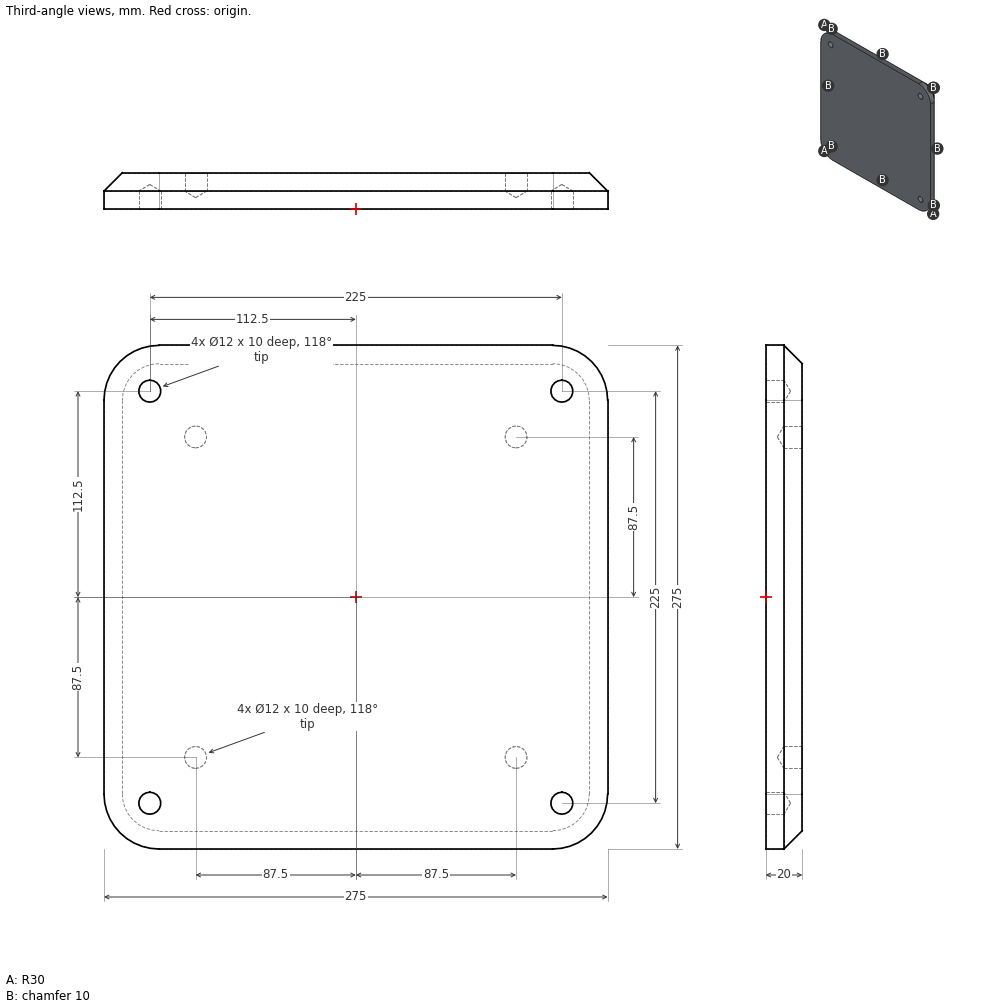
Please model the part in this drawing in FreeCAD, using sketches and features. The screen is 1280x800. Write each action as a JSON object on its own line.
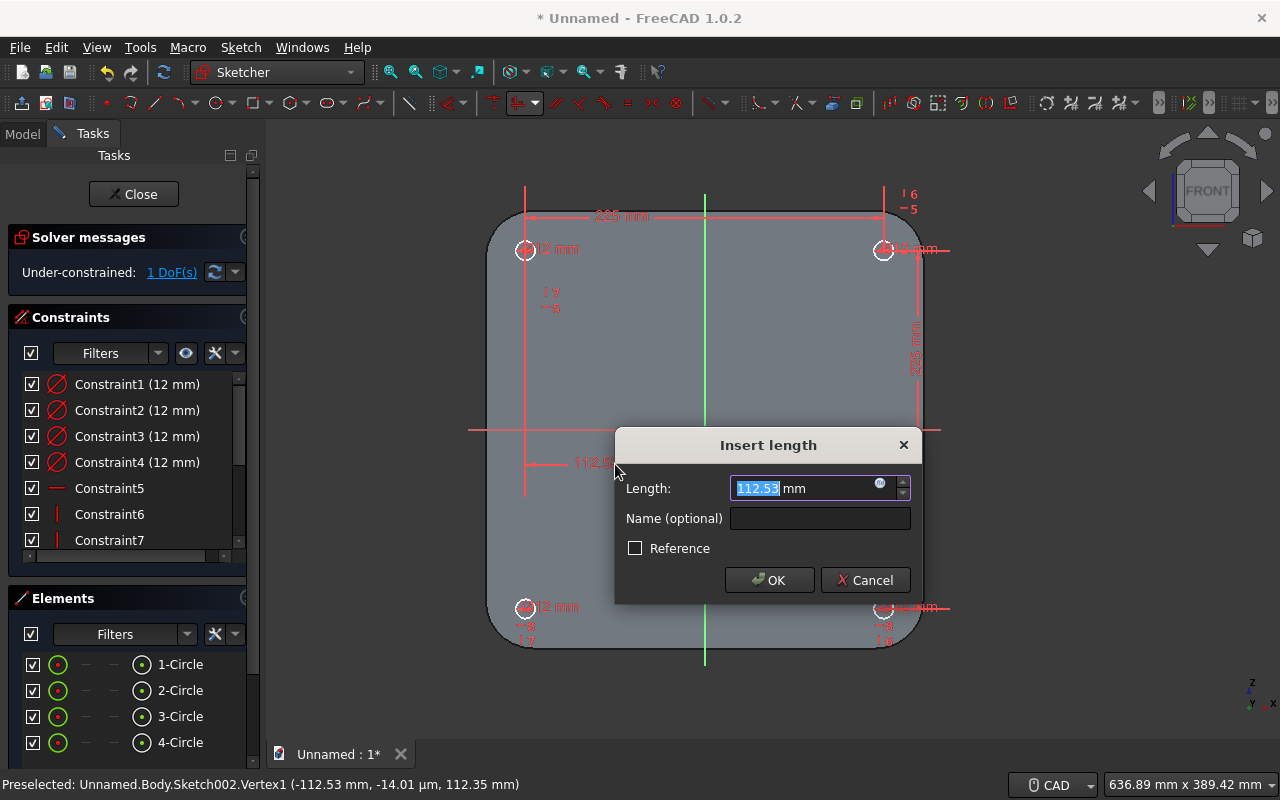
{"action": "type", "text": "112.5"}
{"action": "key", "text": "Return"}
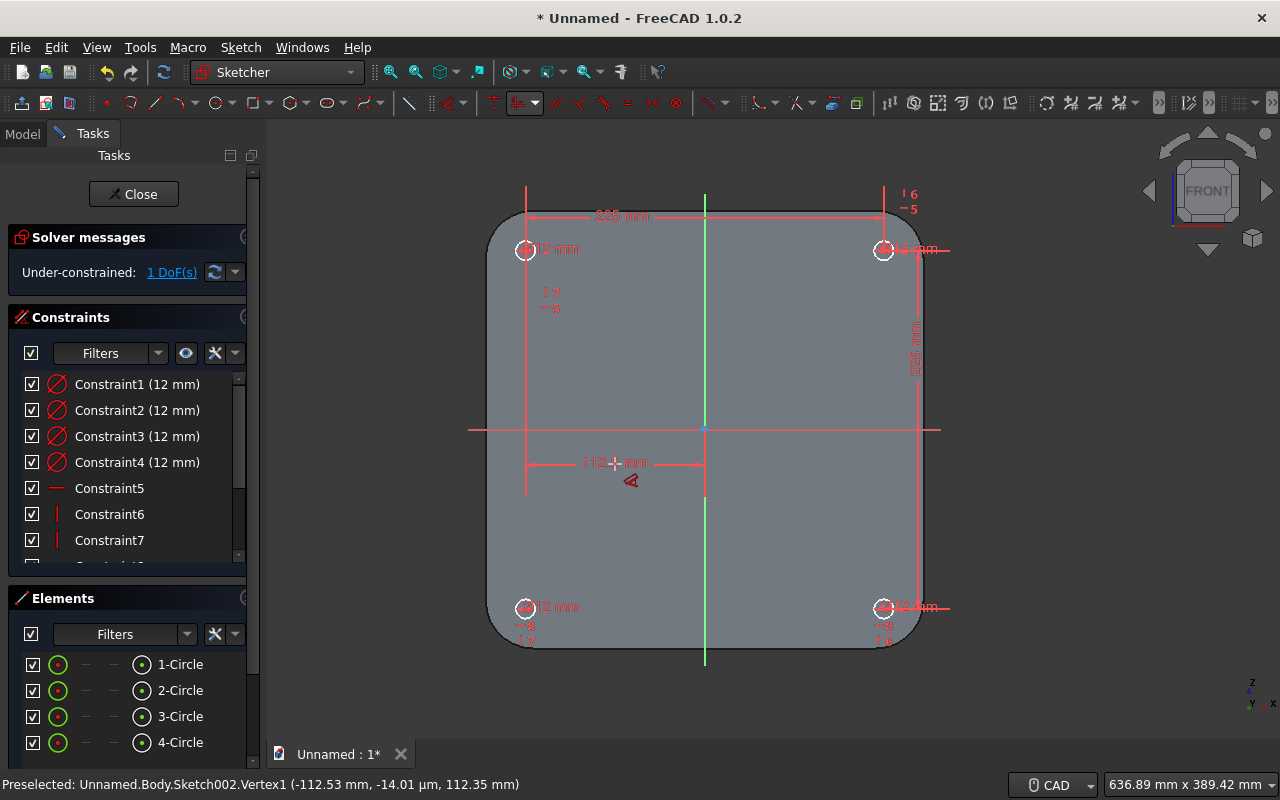
{"action": "left_click", "coordinate": [526, 251]}
{"action": "left_click", "coordinate": [492, 340]}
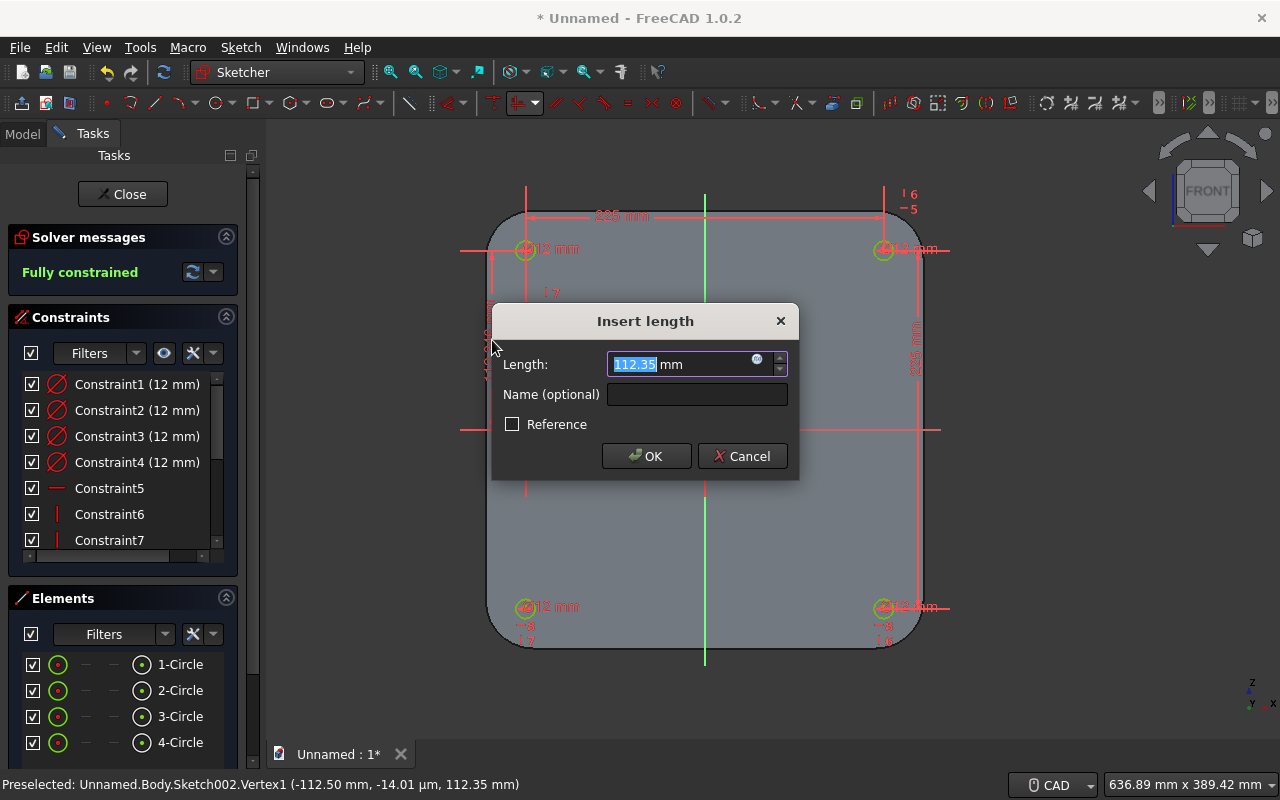
{"action": "type", "text": "112.5"}
{"action": "key", "text": "Return"}
{"action": "key", "text": "Escape"}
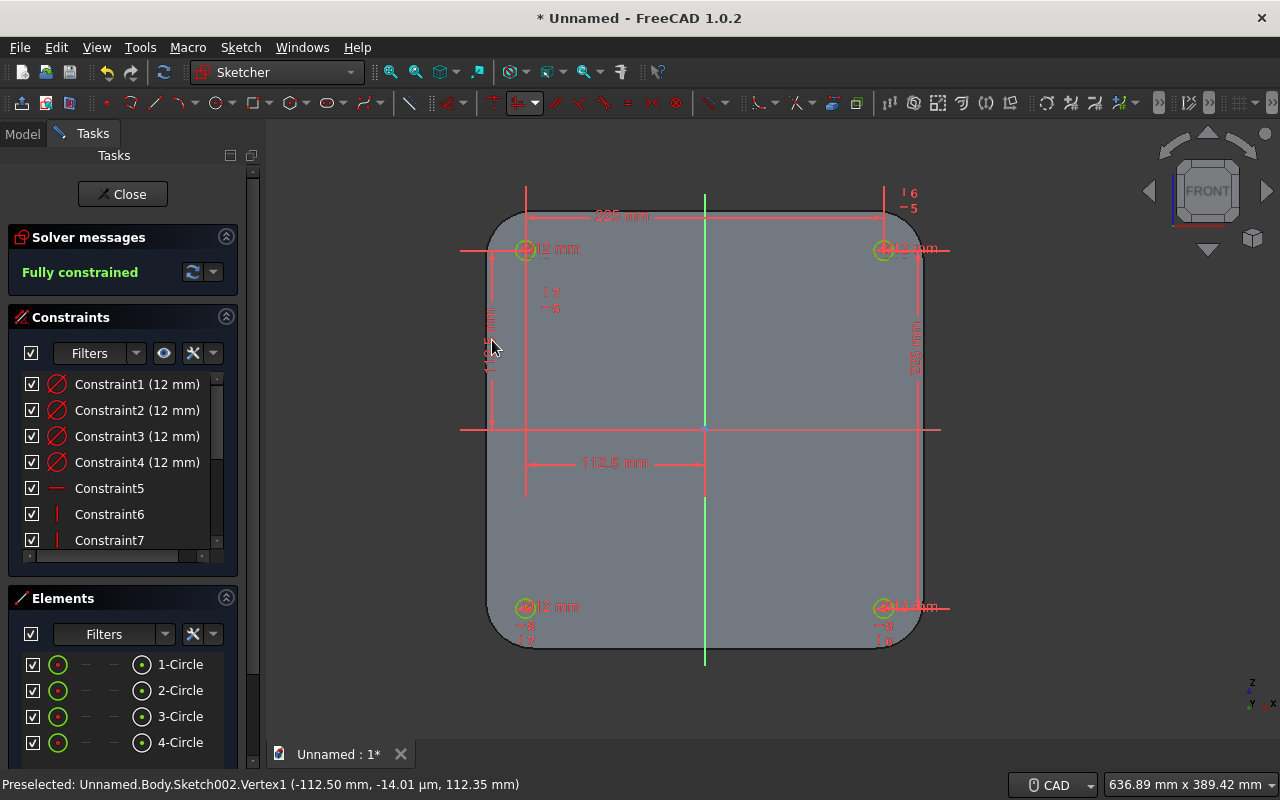
{"action": "left_click", "coordinate": [123, 194]}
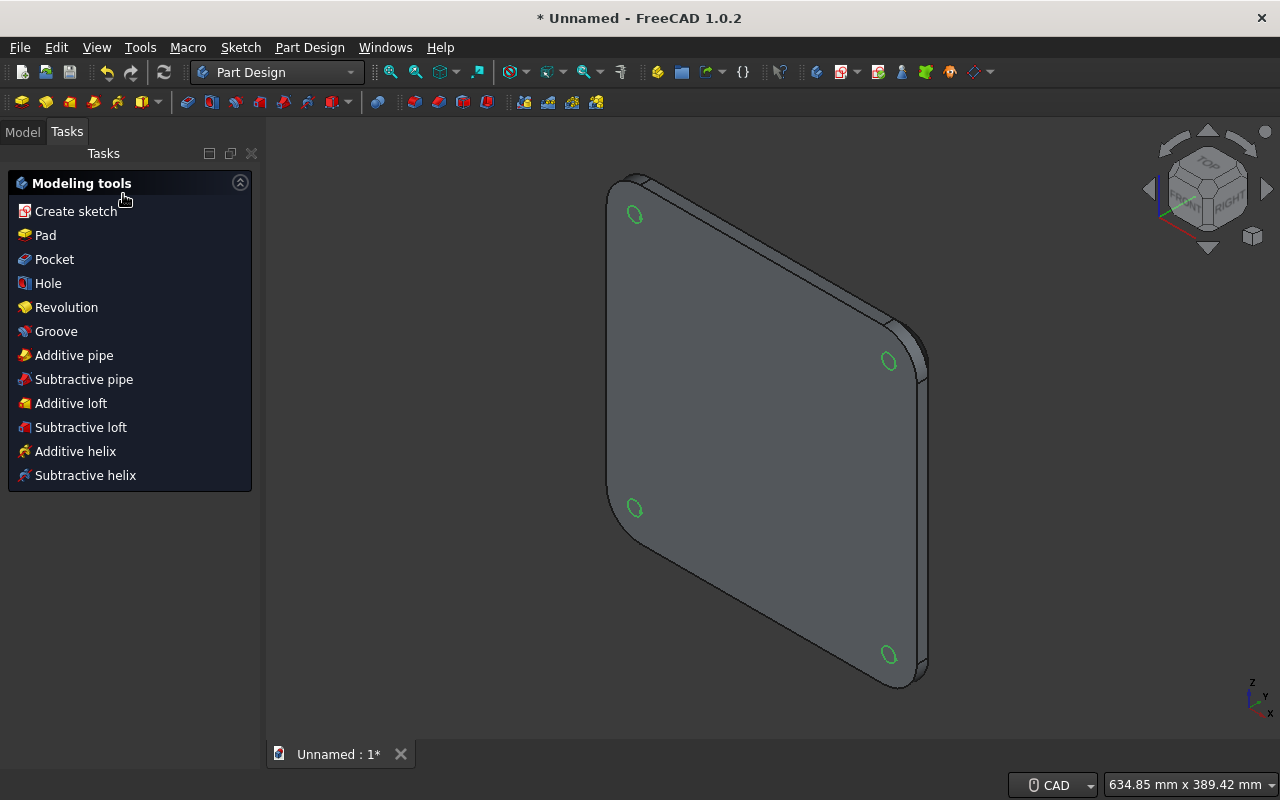
{"action": "left_click", "coordinate": [212, 102]}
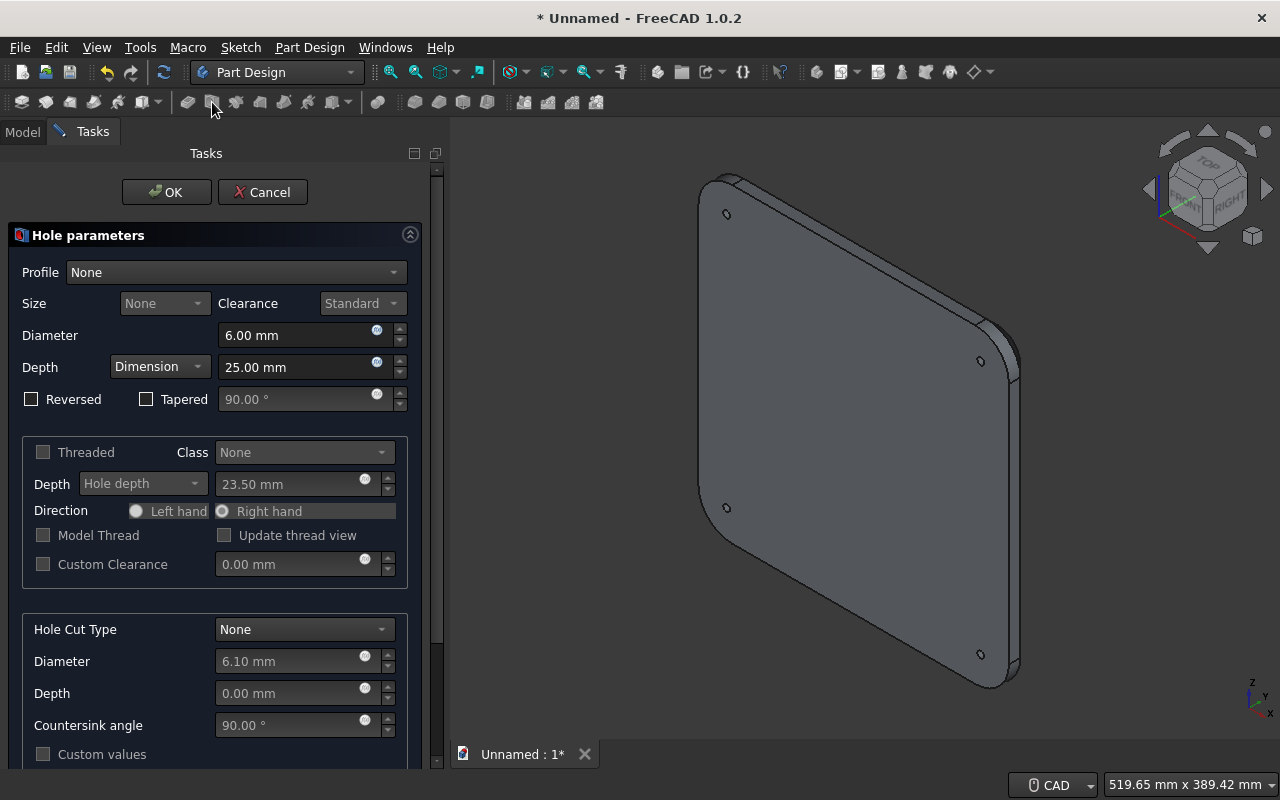
{"action": "triple_click", "coordinate": [305, 335]}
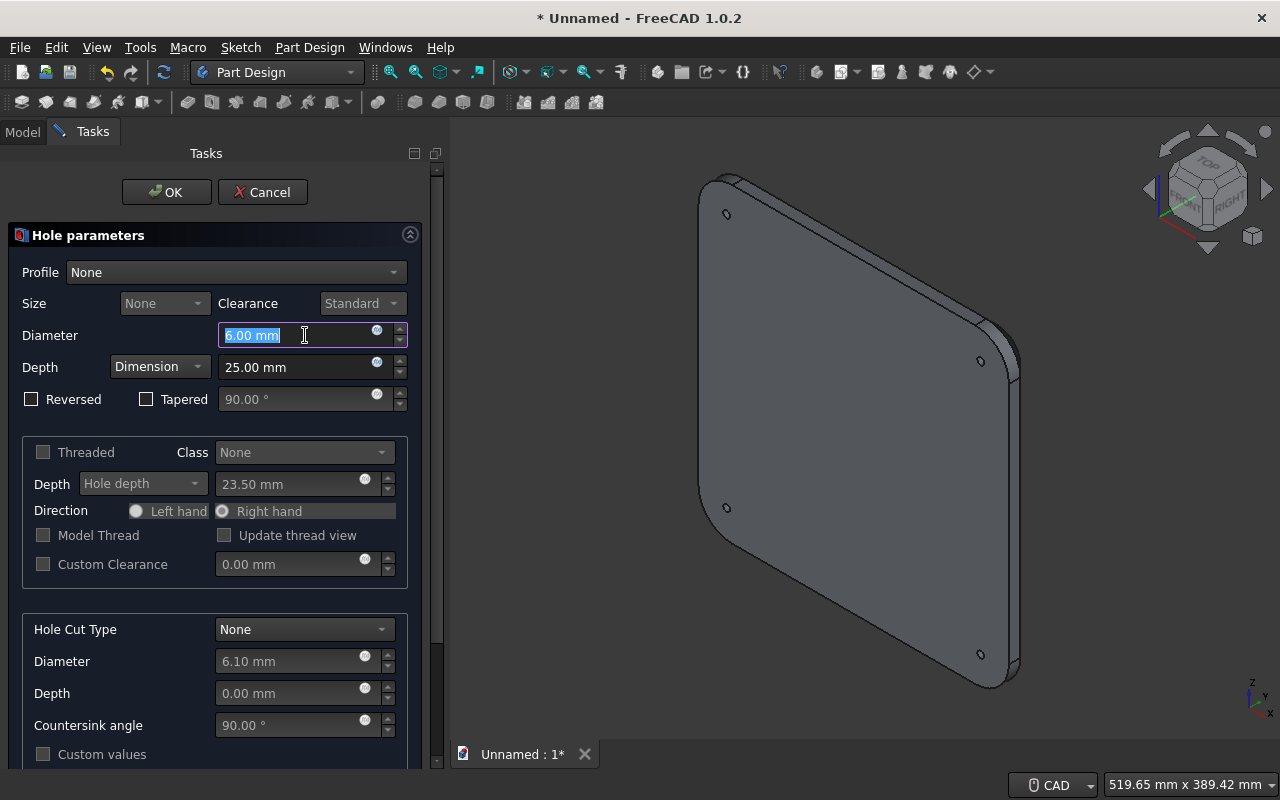
{"action": "type", "text": "12"}
{"action": "key", "text": "Tab"}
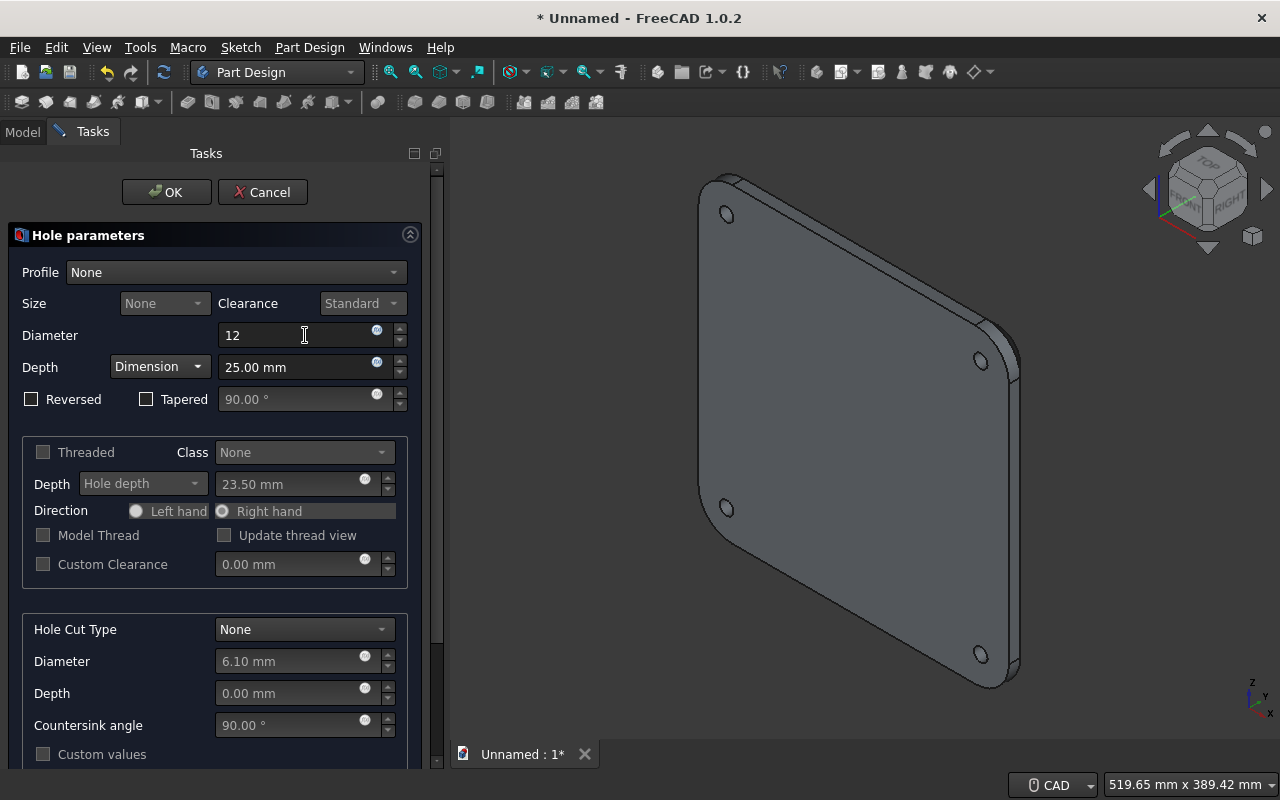
{"action": "triple_click", "coordinate": [305, 367]}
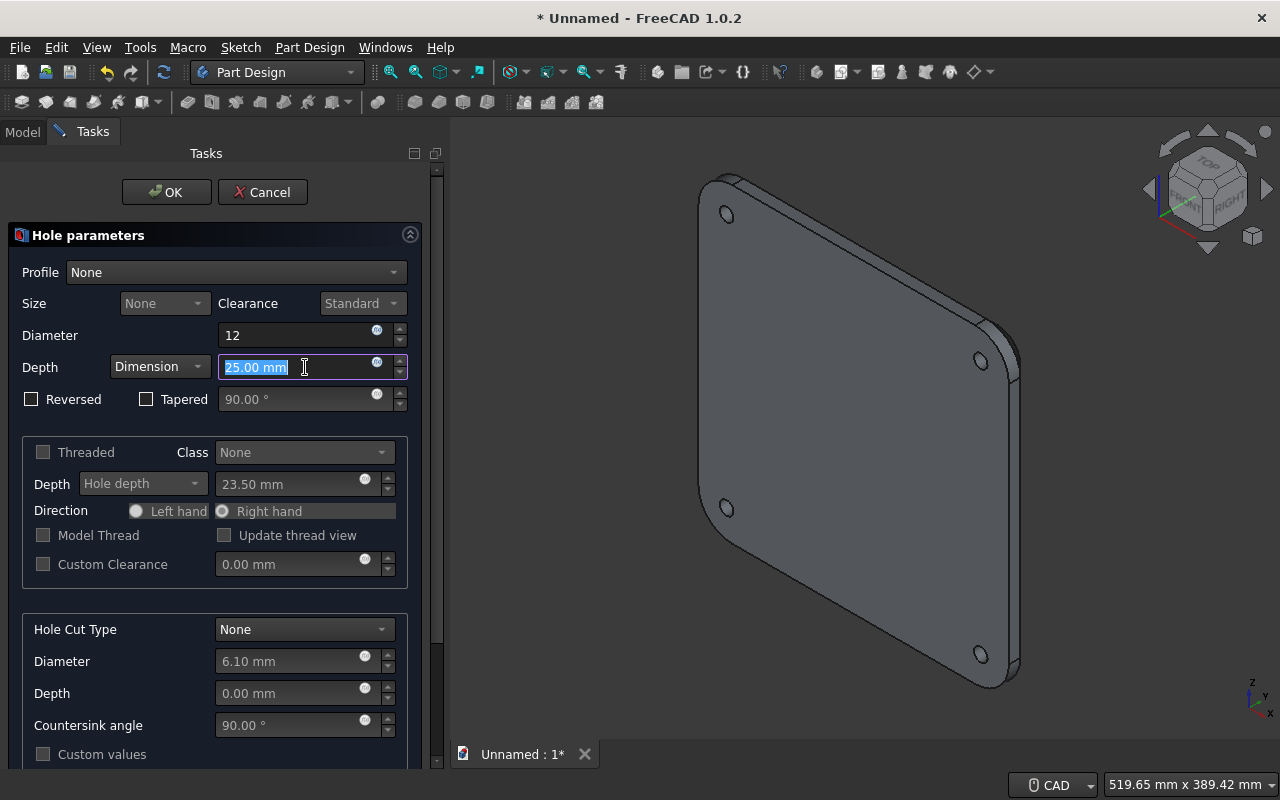
{"action": "type", "text": "10"}
{"action": "key", "text": "Tab"}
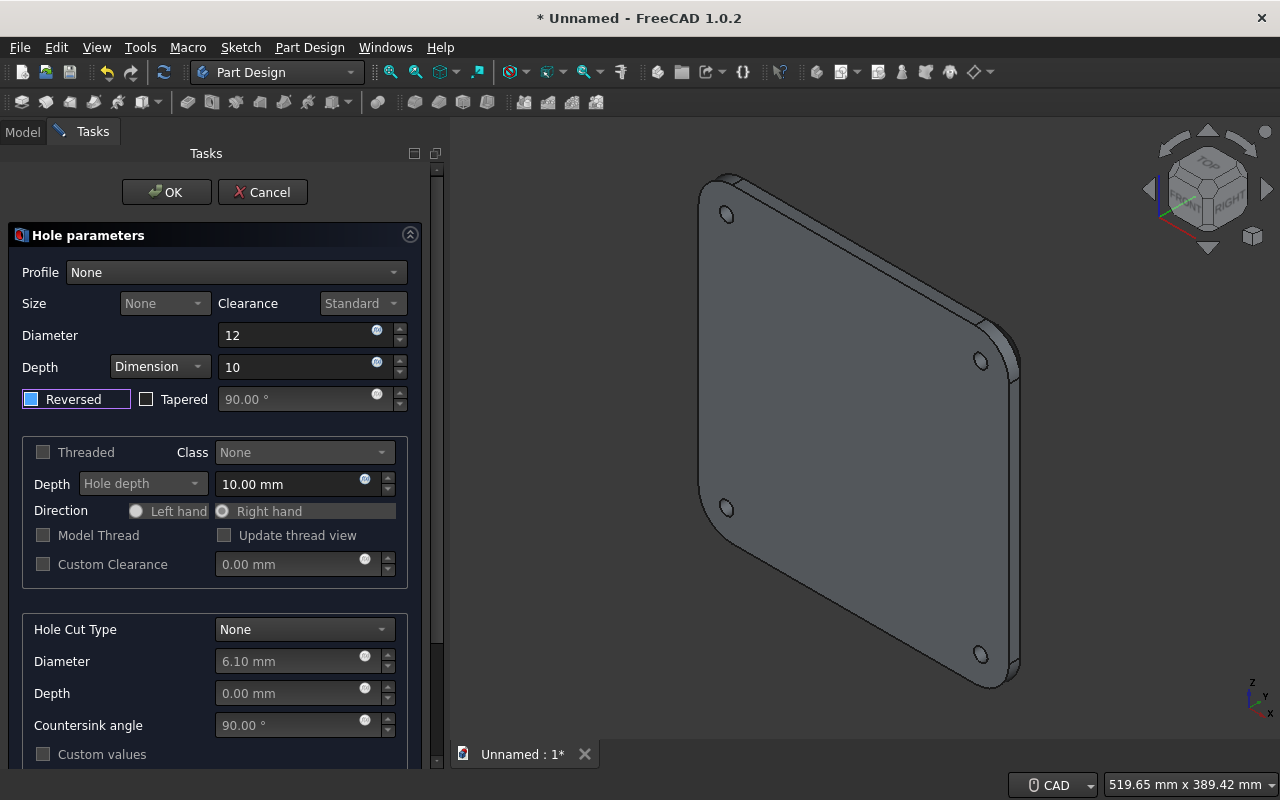
{"action": "left_click", "coordinate": [167, 192]}